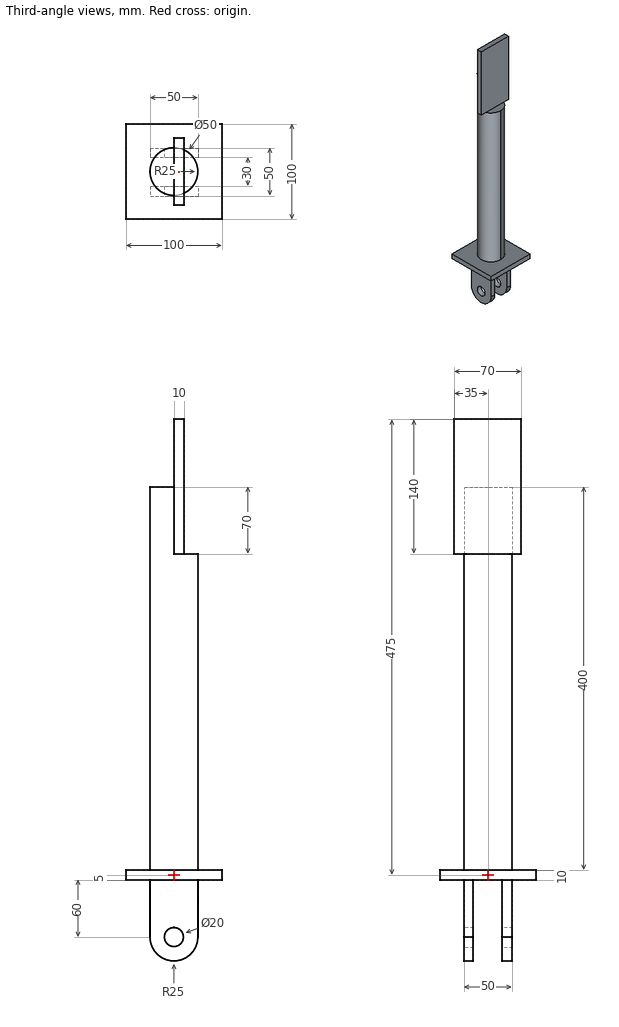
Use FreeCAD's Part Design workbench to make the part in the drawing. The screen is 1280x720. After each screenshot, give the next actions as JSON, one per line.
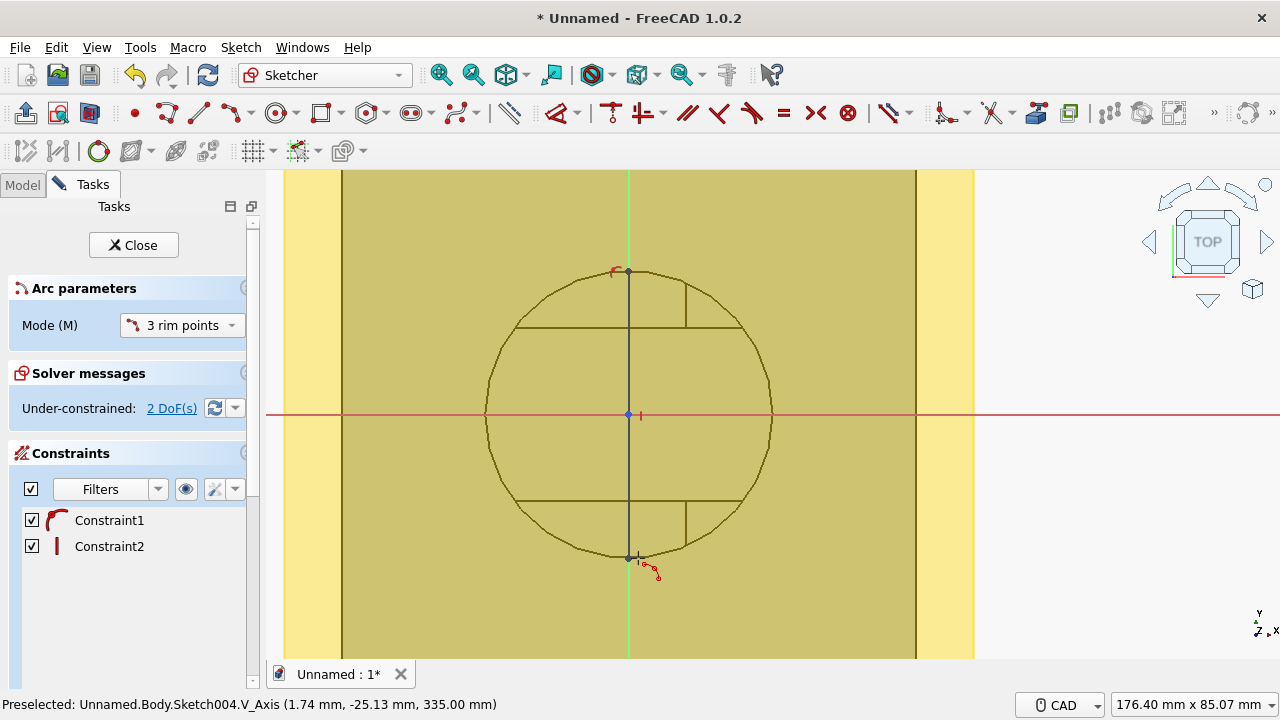
{"action": "left_click", "coordinate": [638, 558]}
{"action": "left_click", "coordinate": [629, 272]}
{"action": "left_click", "coordinate": [766, 459]}
{"action": "key", "text": "Escape"}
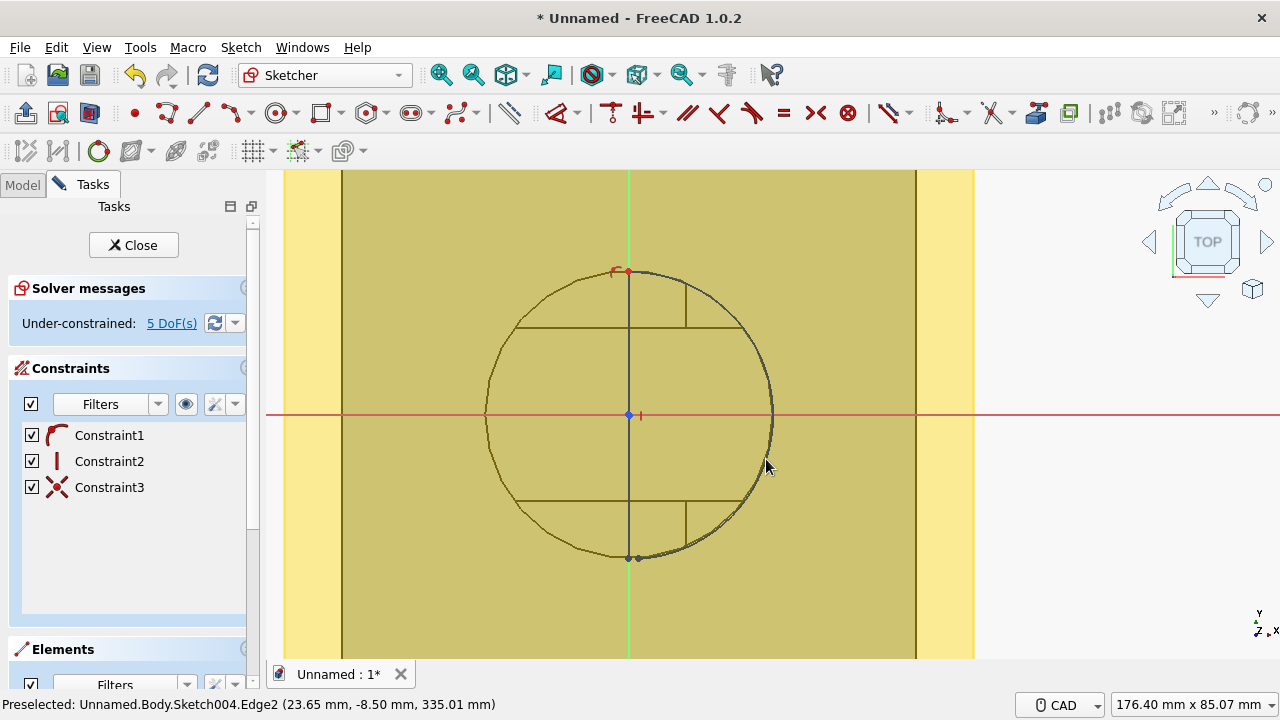
{"action": "left_click_drag", "start_coordinate": [619, 404], "coordinate": [639, 426]}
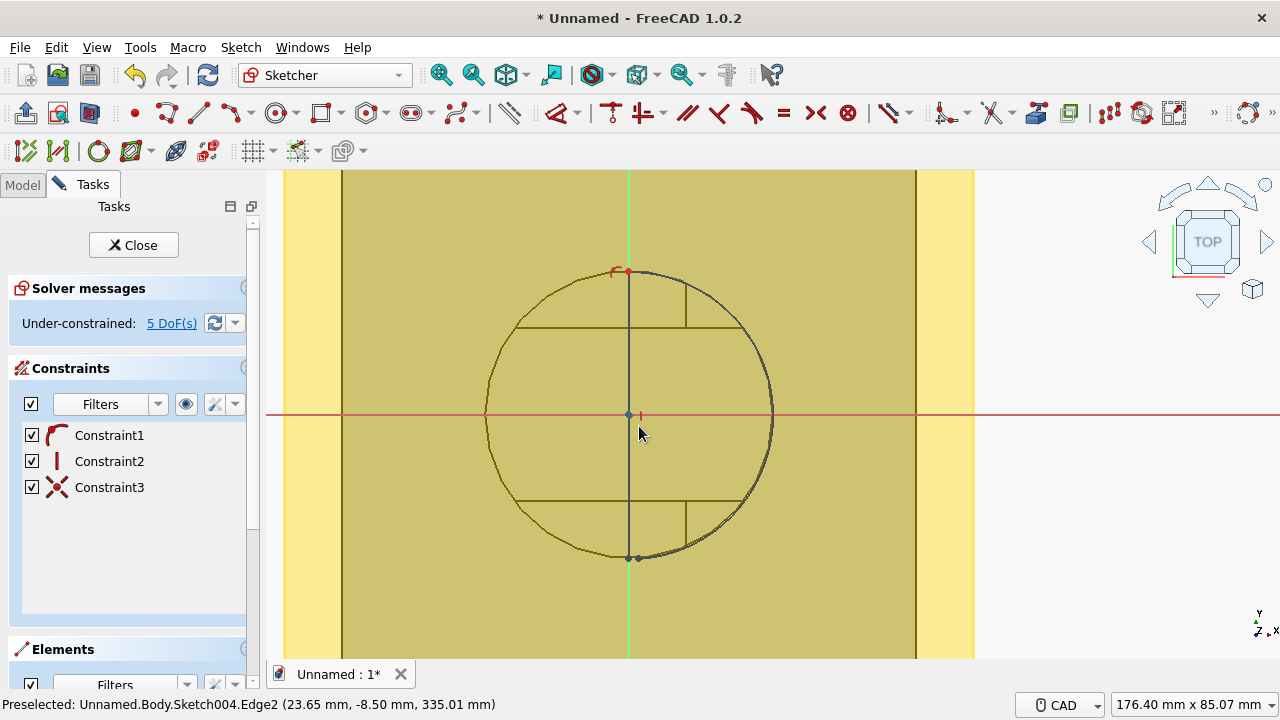
{"action": "key", "text": "c"}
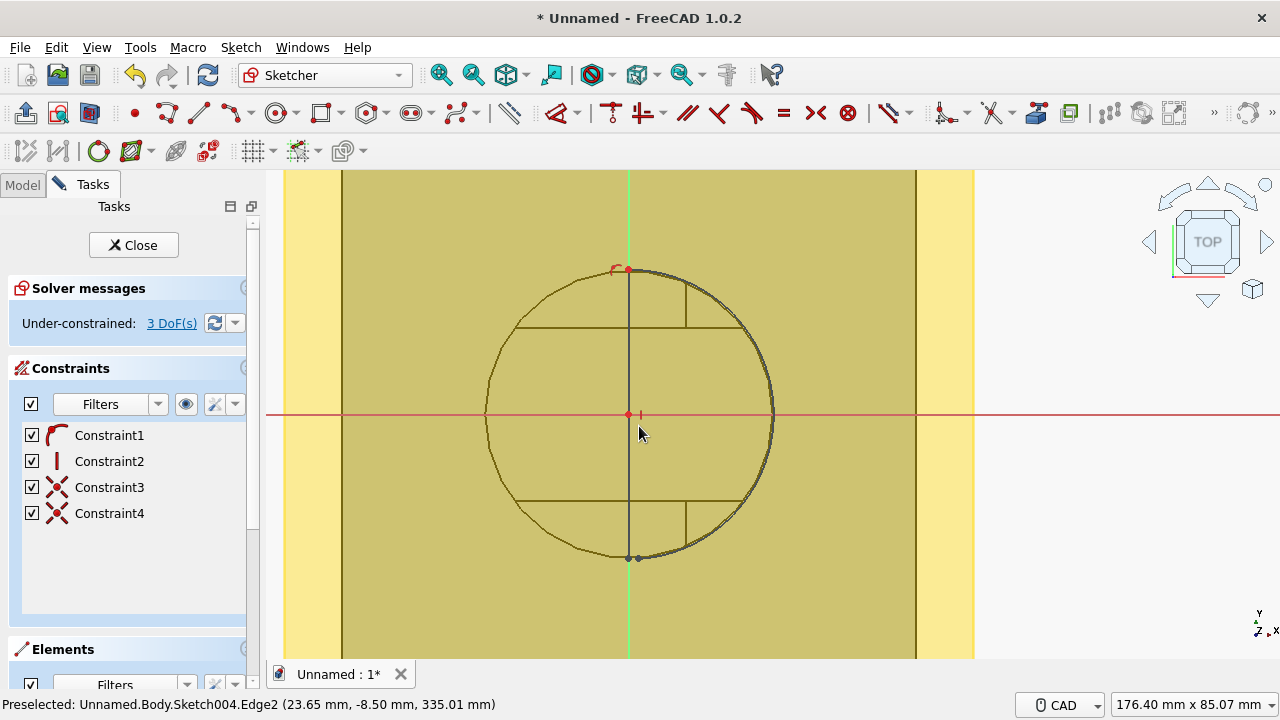
{"action": "key", "text": "d"}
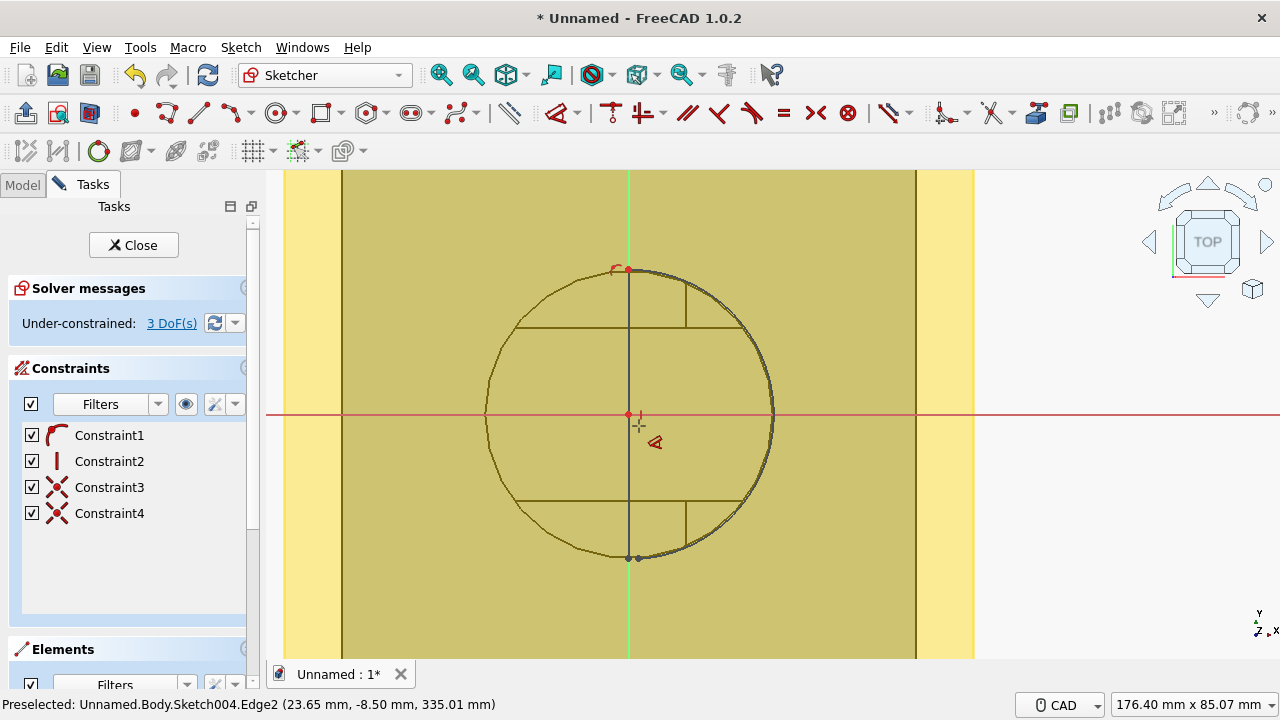
{"action": "left_click", "coordinate": [750, 494]}
{"action": "left_click", "coordinate": [777, 512]}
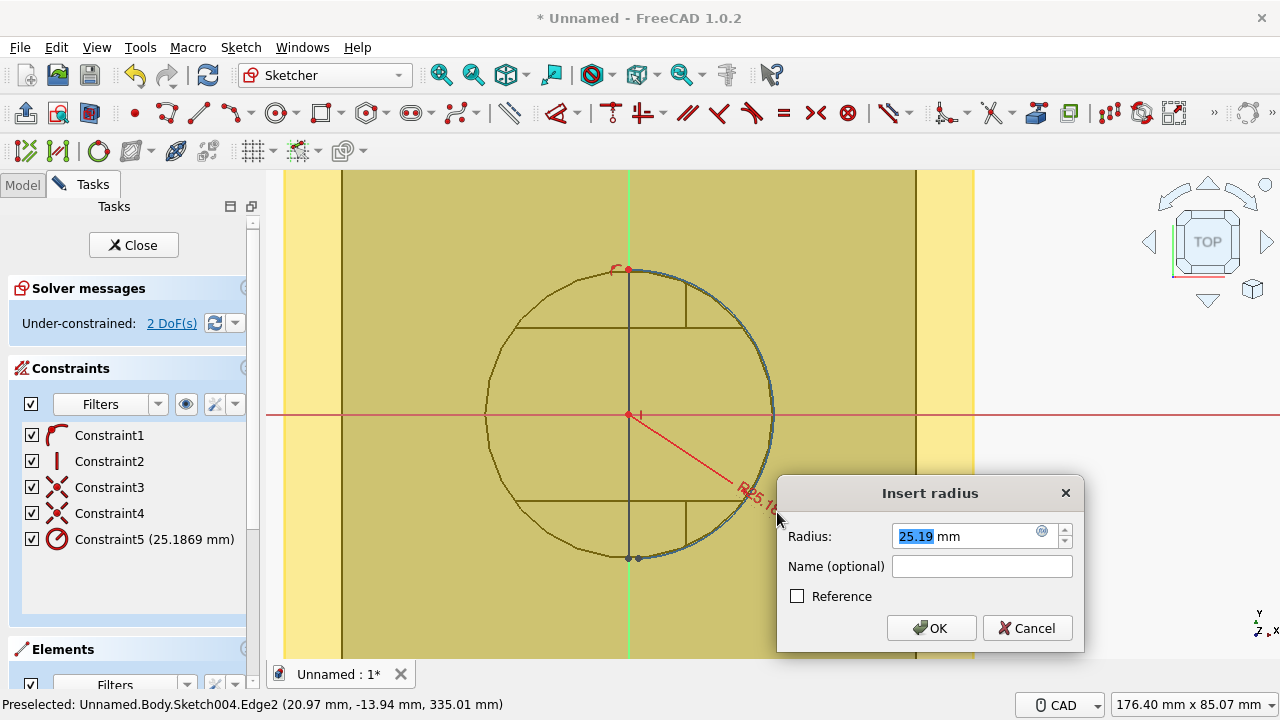
{"action": "type", "text": "25"}
{"action": "key", "text": "Return"}
{"action": "key", "text": "Escape"}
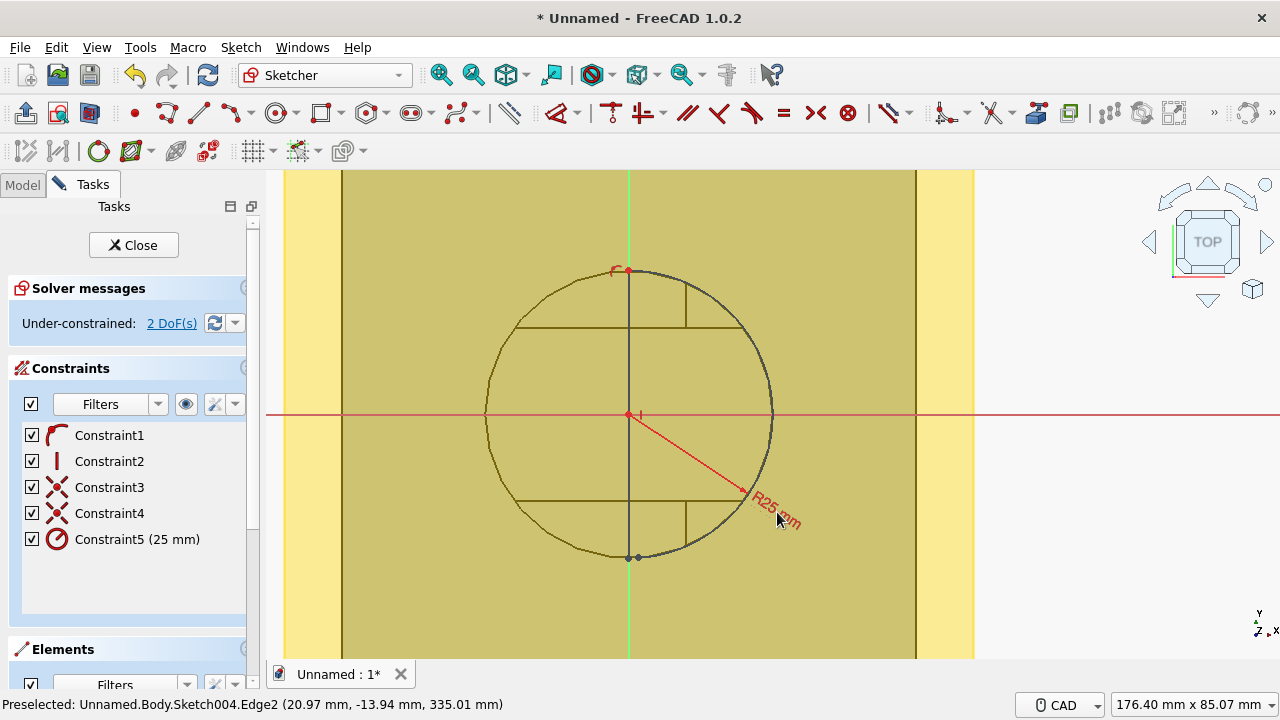
{"action": "left_click", "coordinate": [638, 558]}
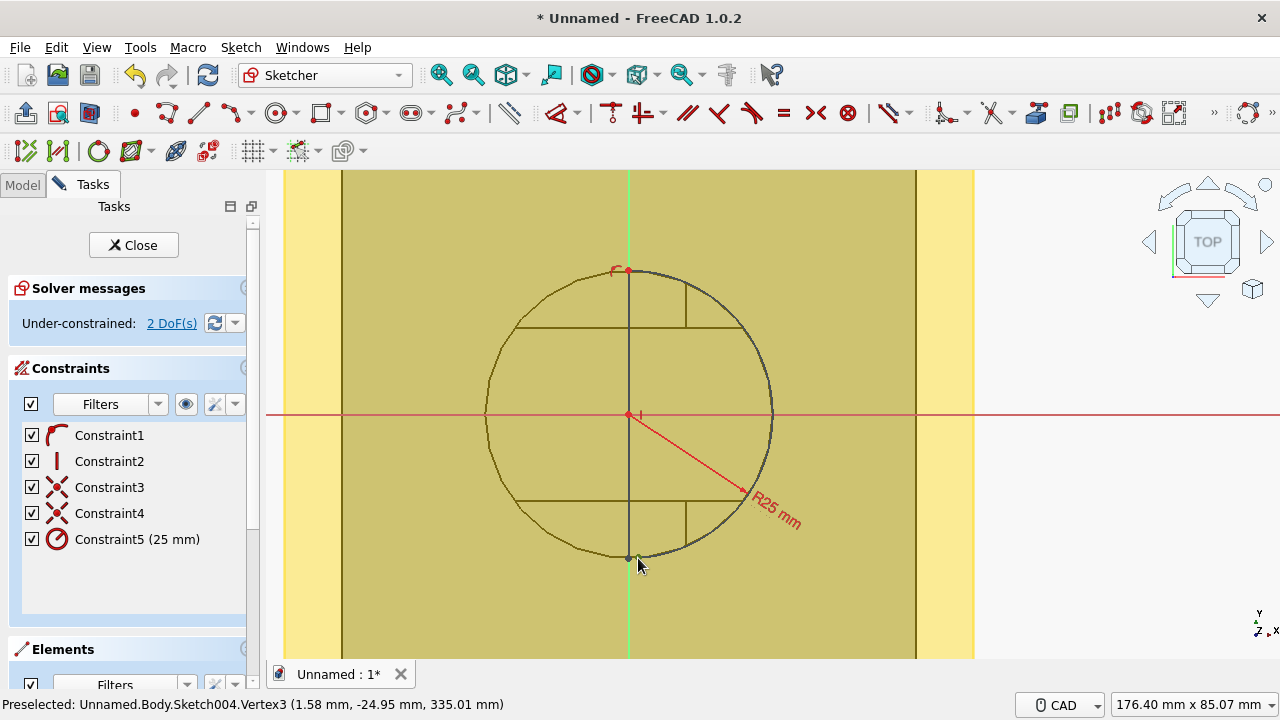
{"action": "left_click", "coordinate": [629, 600]}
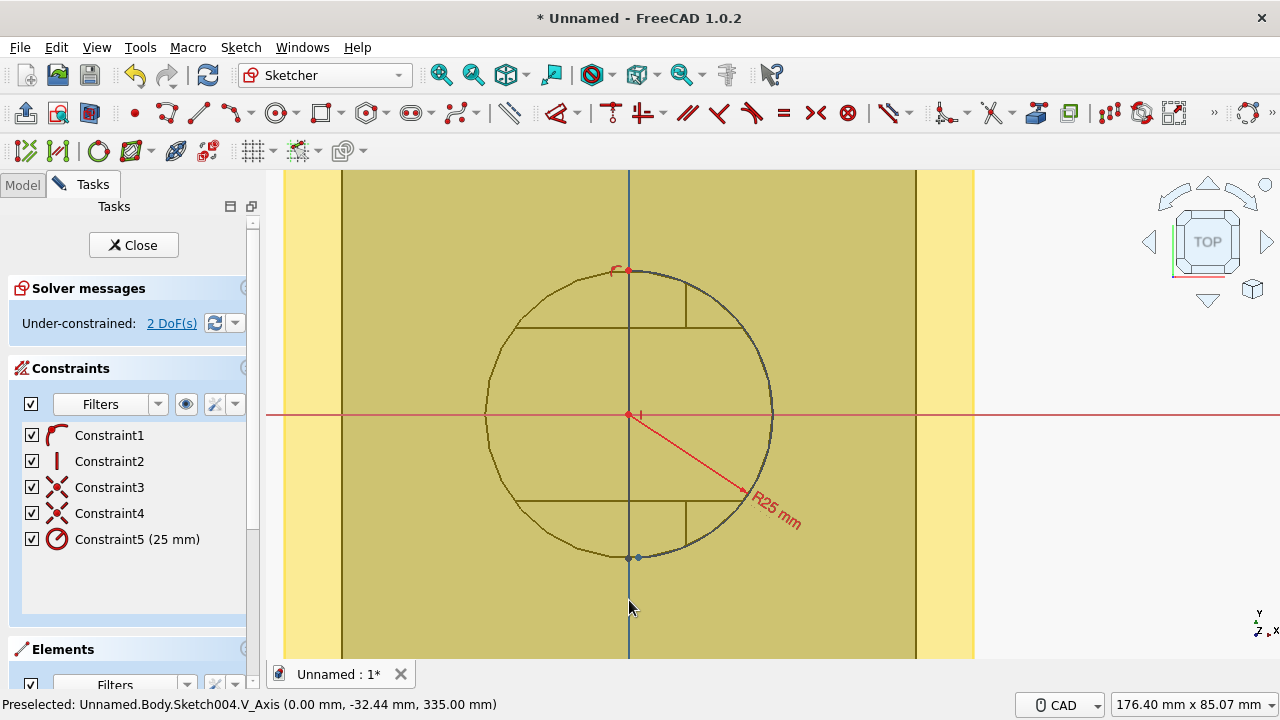
{"action": "left_click", "coordinate": [612, 114]}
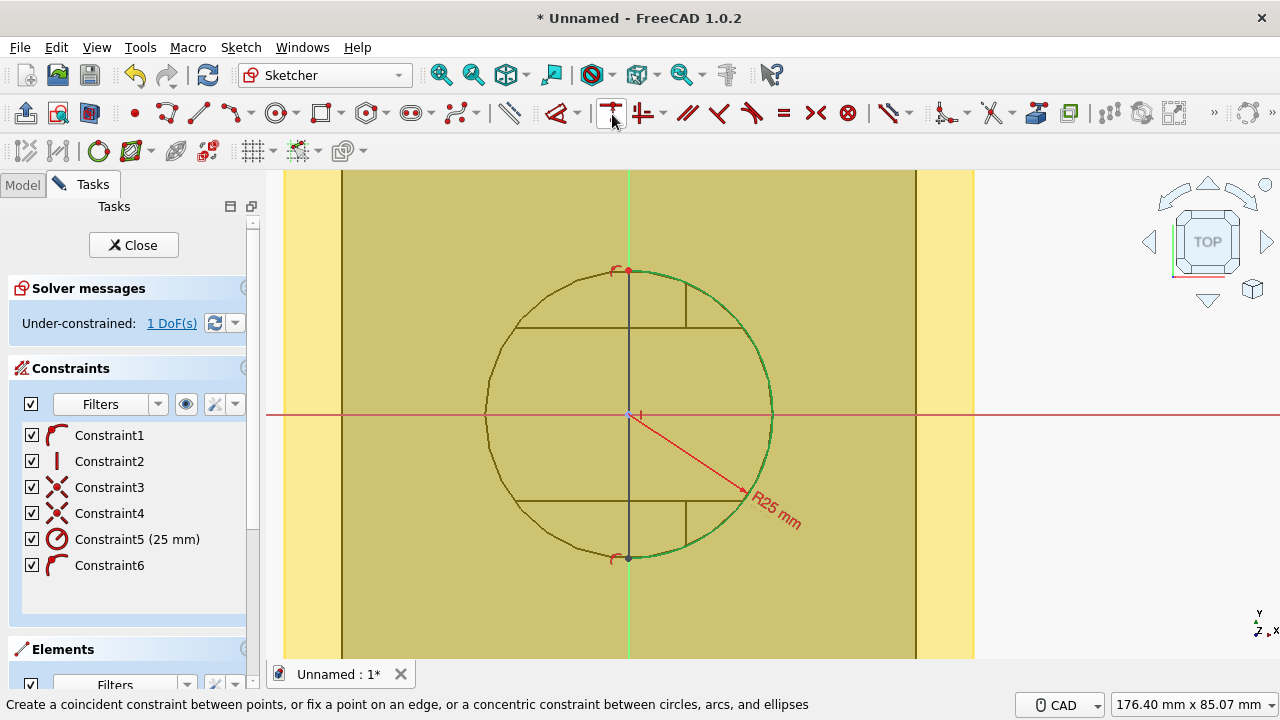
{"action": "left_click", "coordinate": [556, 114]}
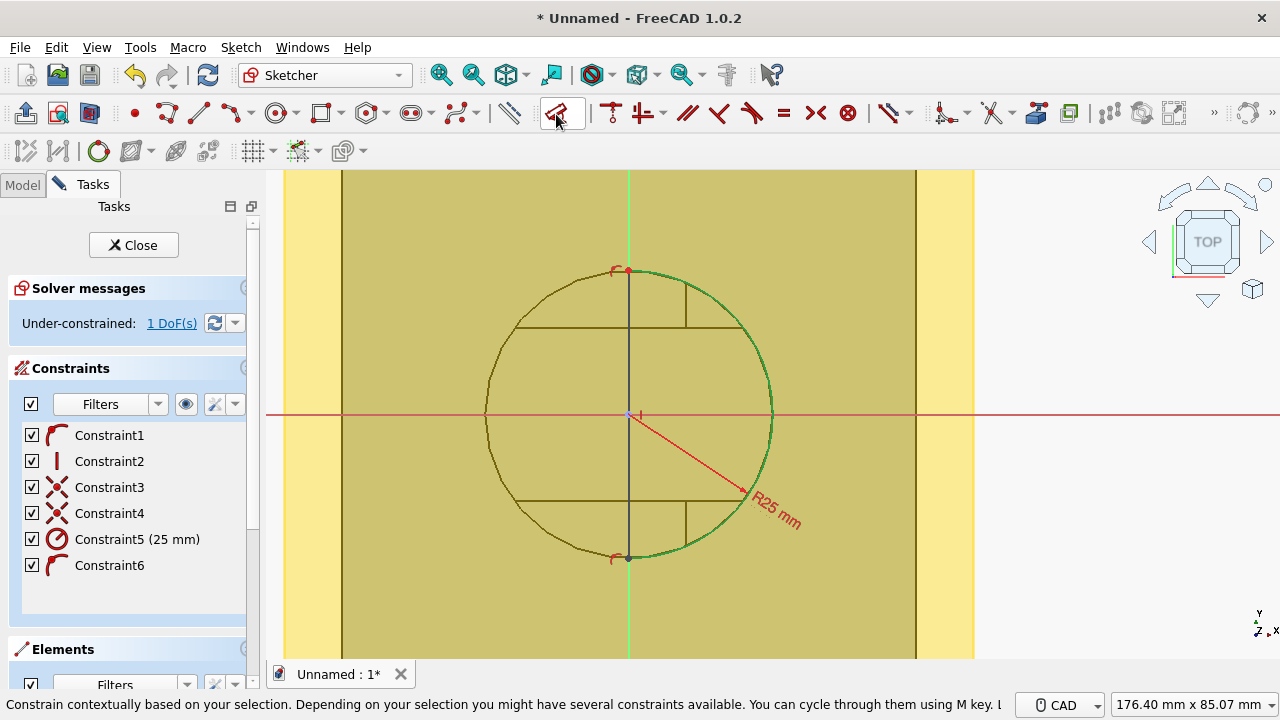
{"action": "left_click", "coordinate": [629, 357]}
{"action": "left_click", "coordinate": [595, 349]}